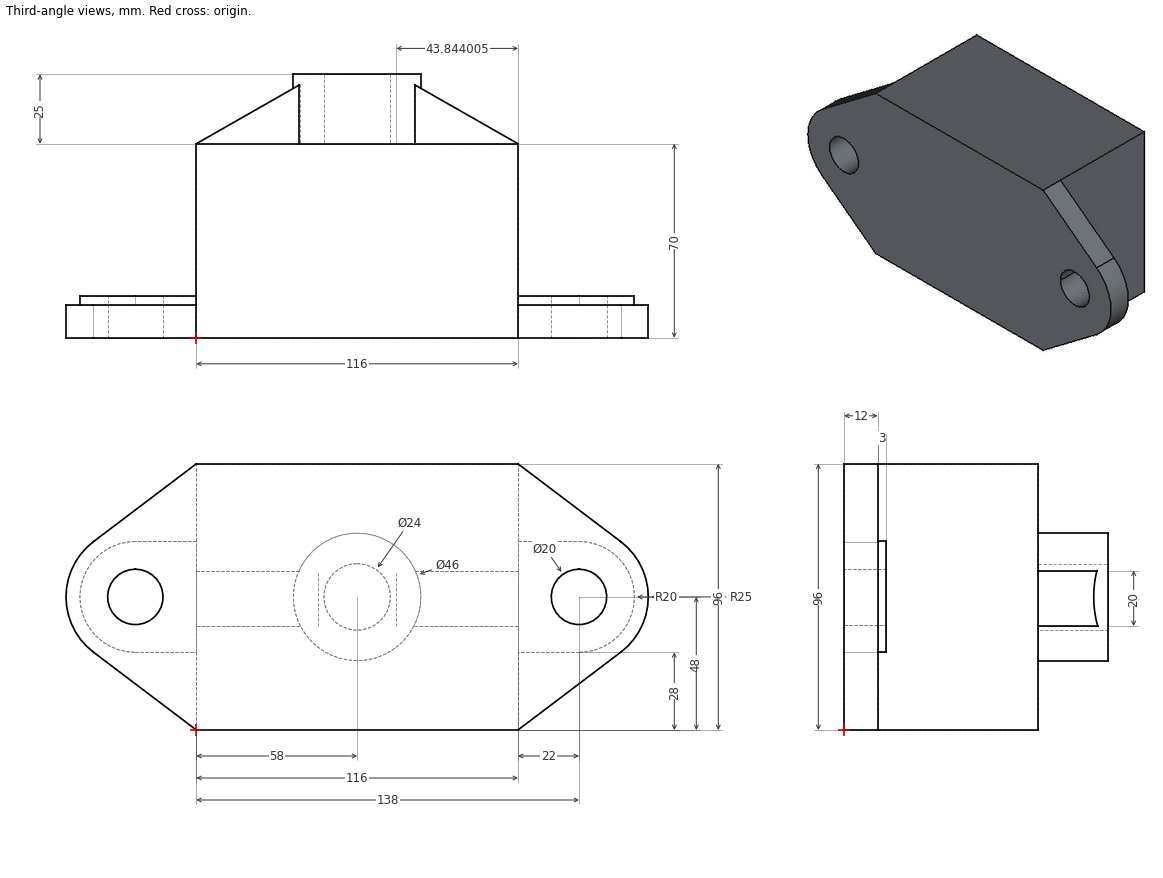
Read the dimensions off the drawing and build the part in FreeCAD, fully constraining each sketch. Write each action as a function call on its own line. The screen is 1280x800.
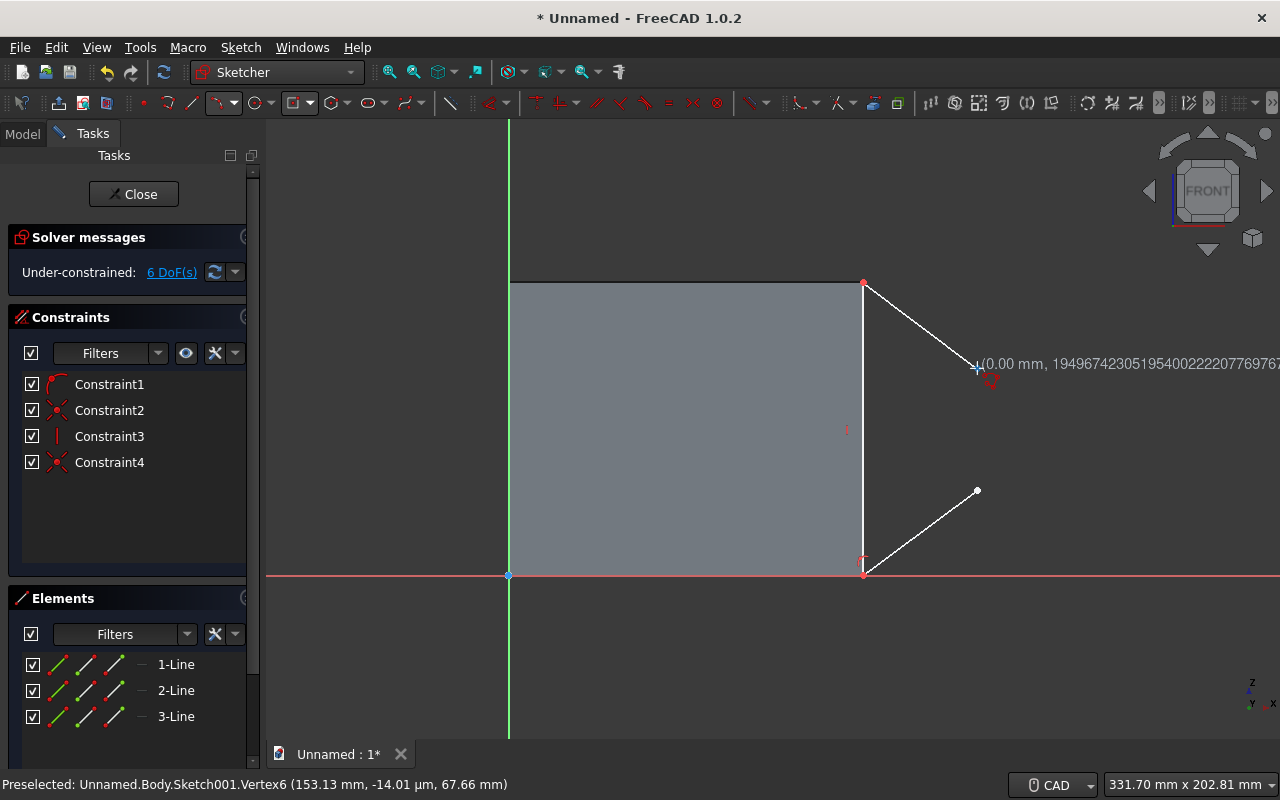
click(218, 104)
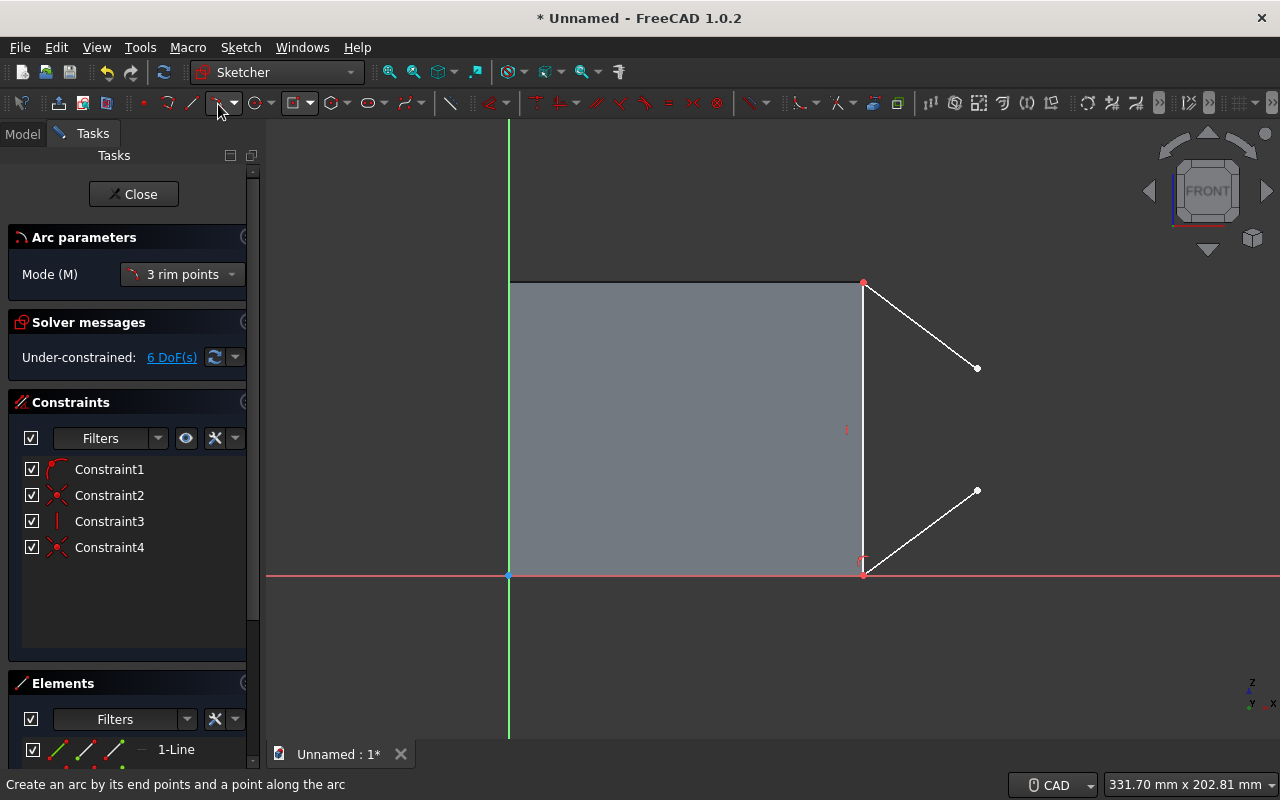
click(977, 369)
click(977, 491)
click(1007, 429)
key(Escape)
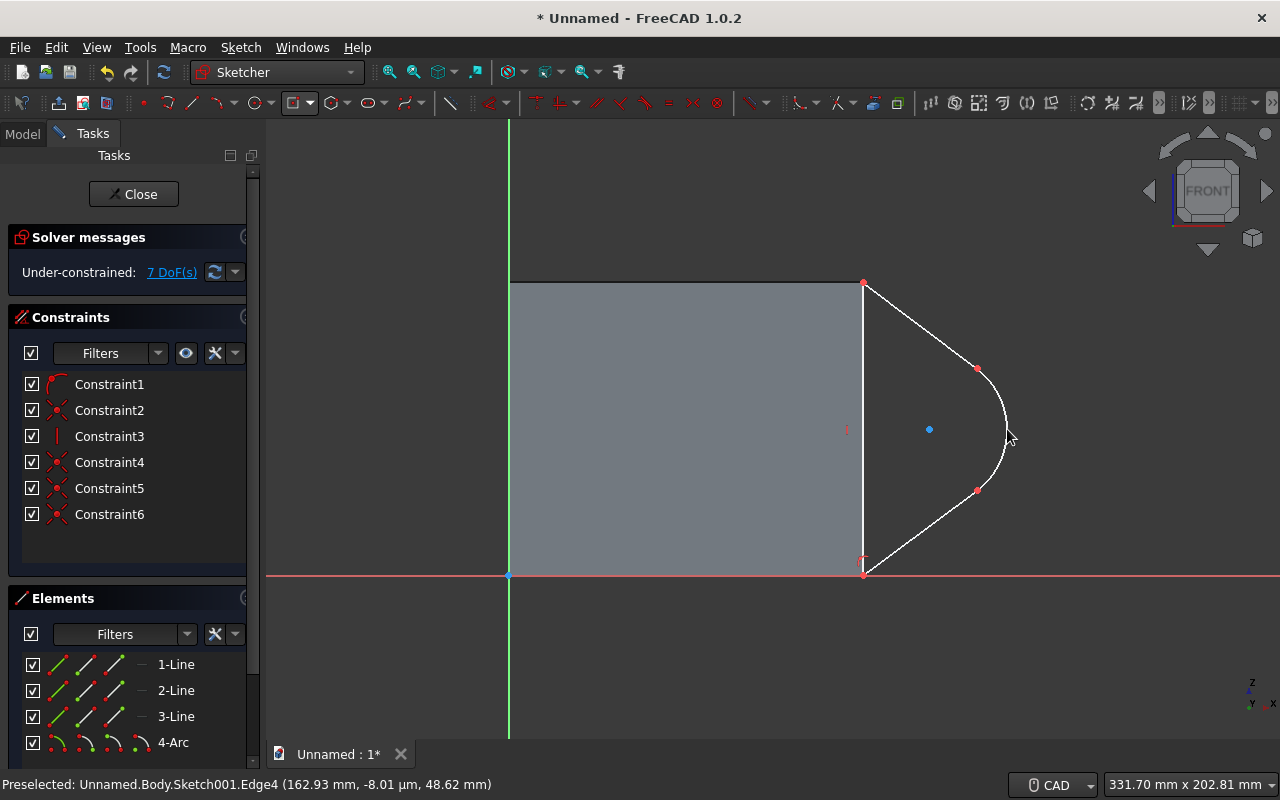
click(943, 516)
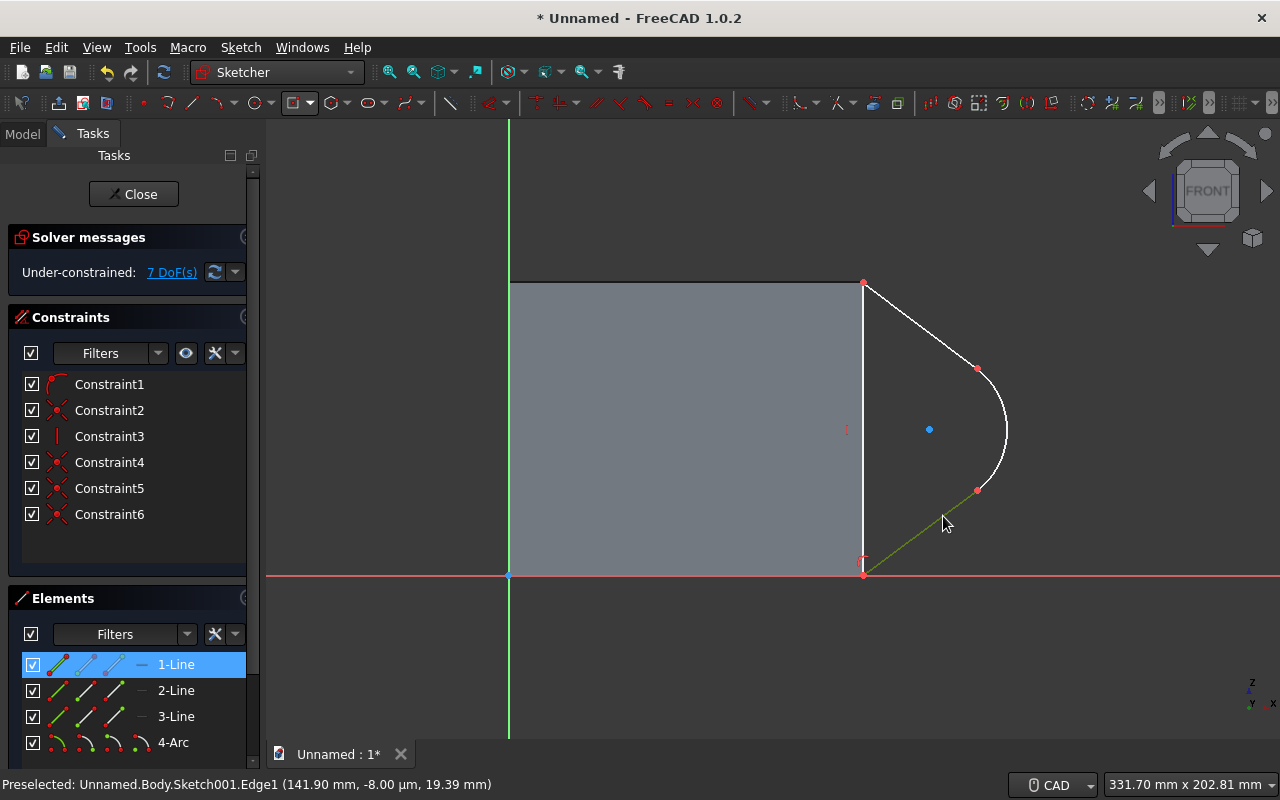
click(1002, 458)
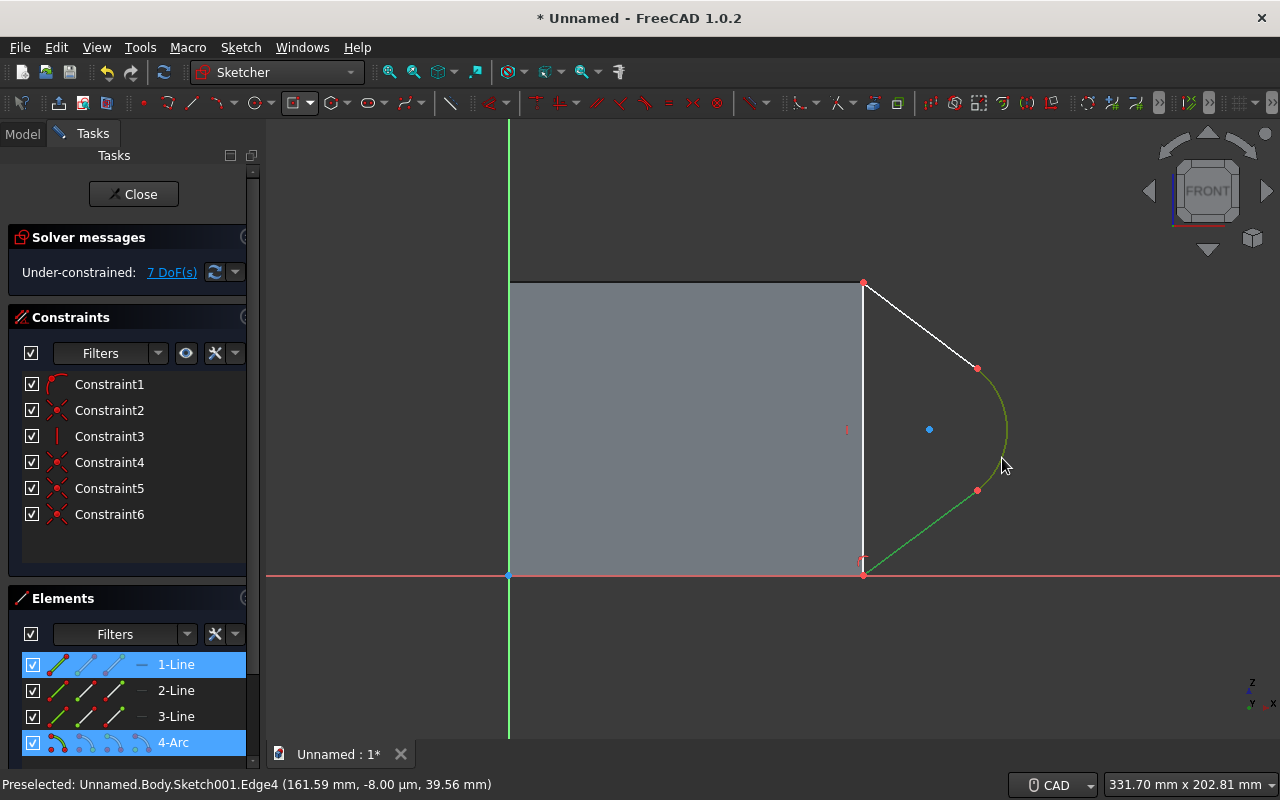
click(646, 104)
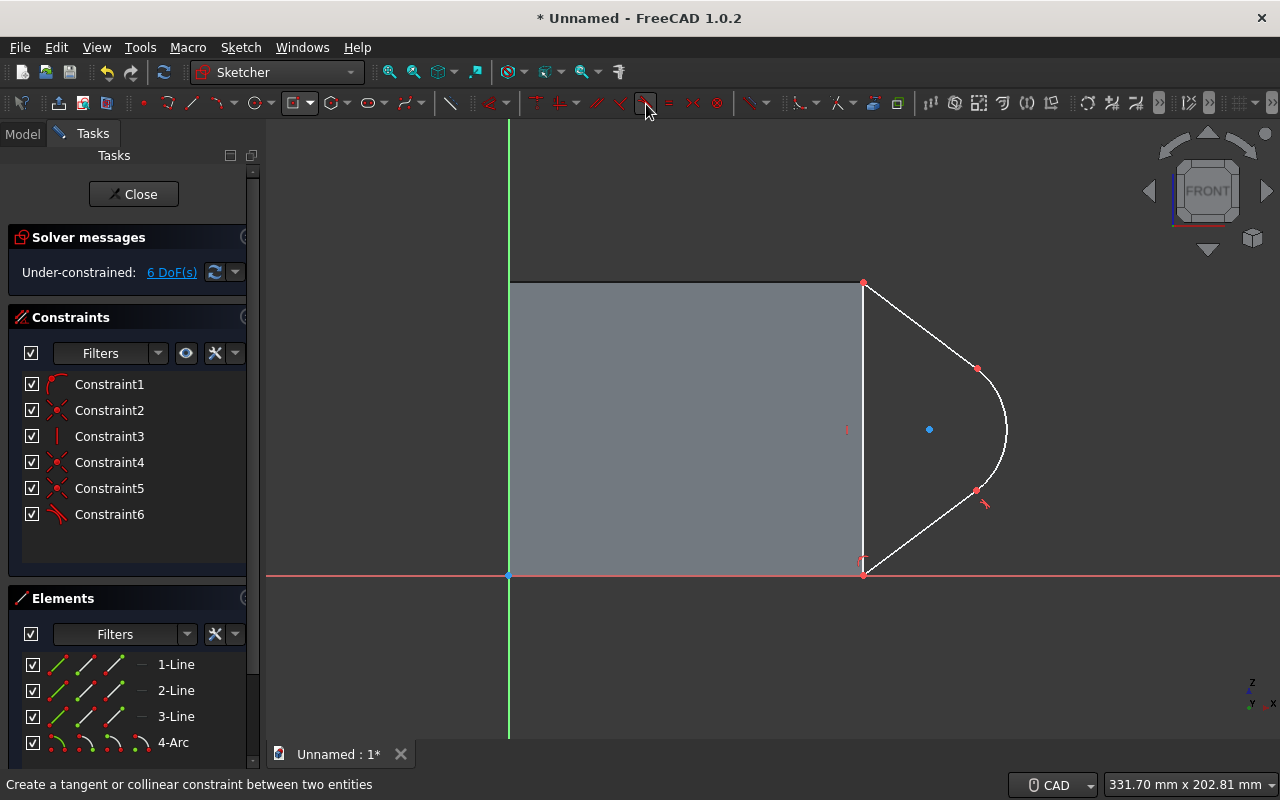
click(897, 309)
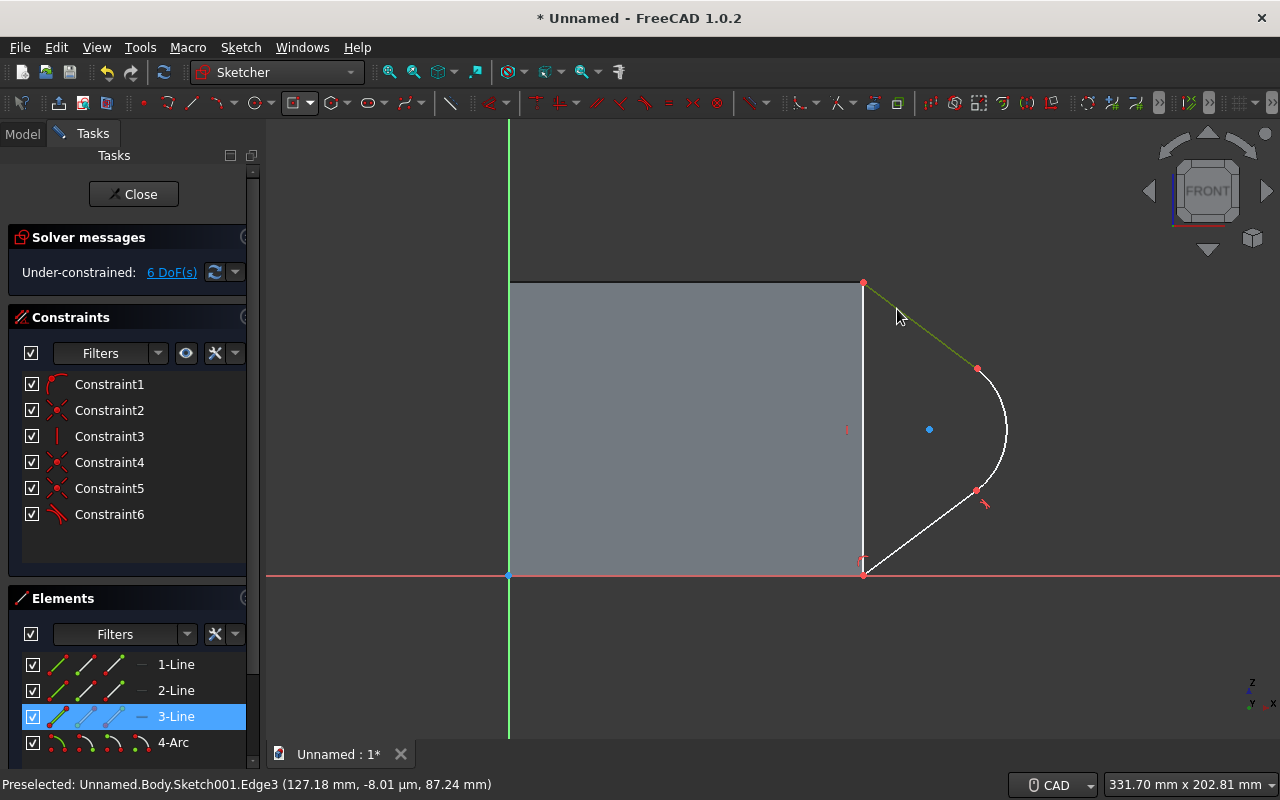
click(1001, 458)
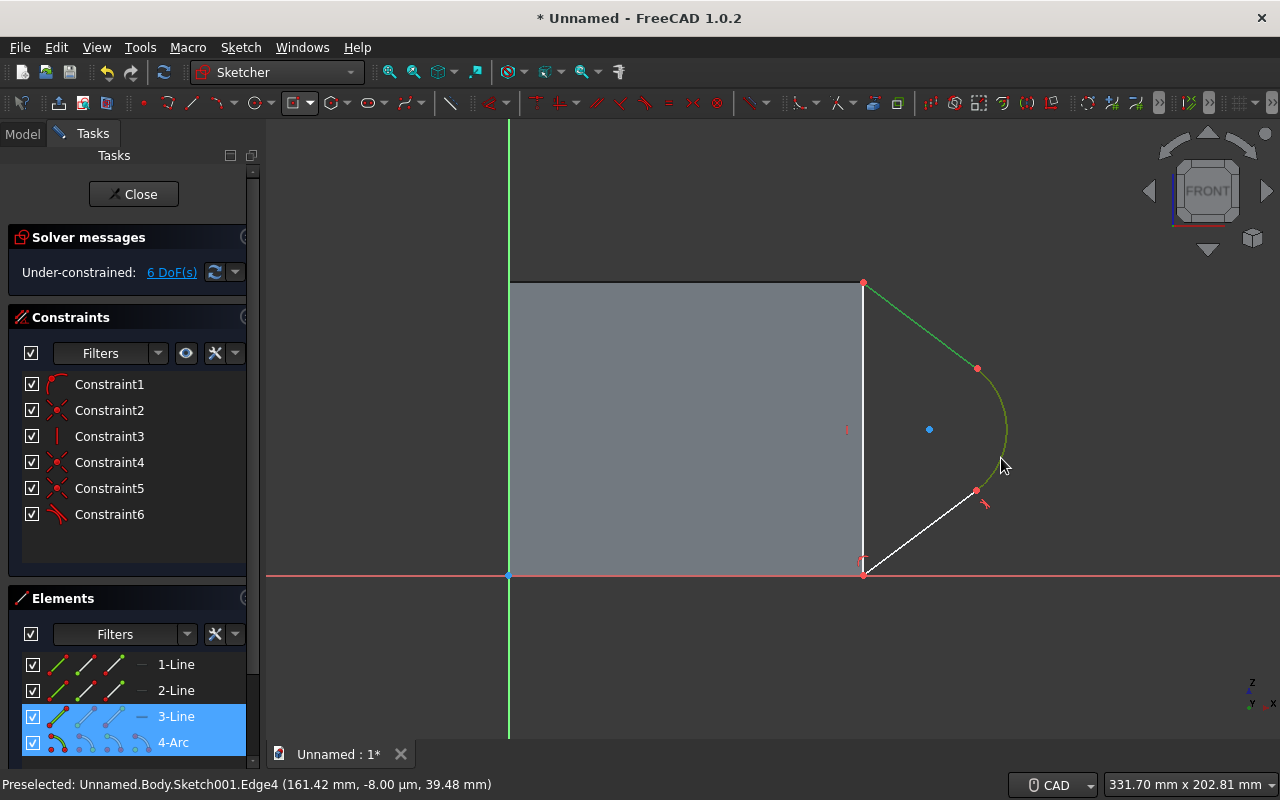
click(646, 104)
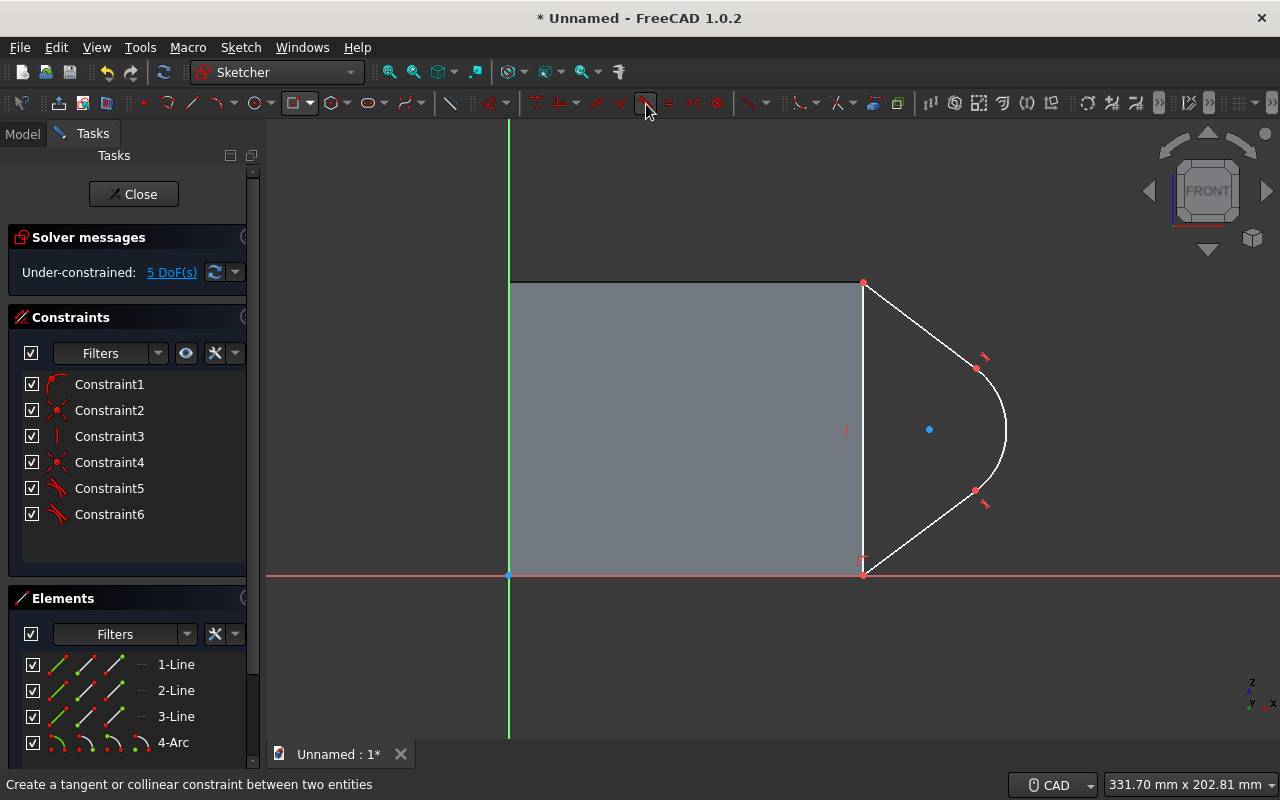
click(490, 104)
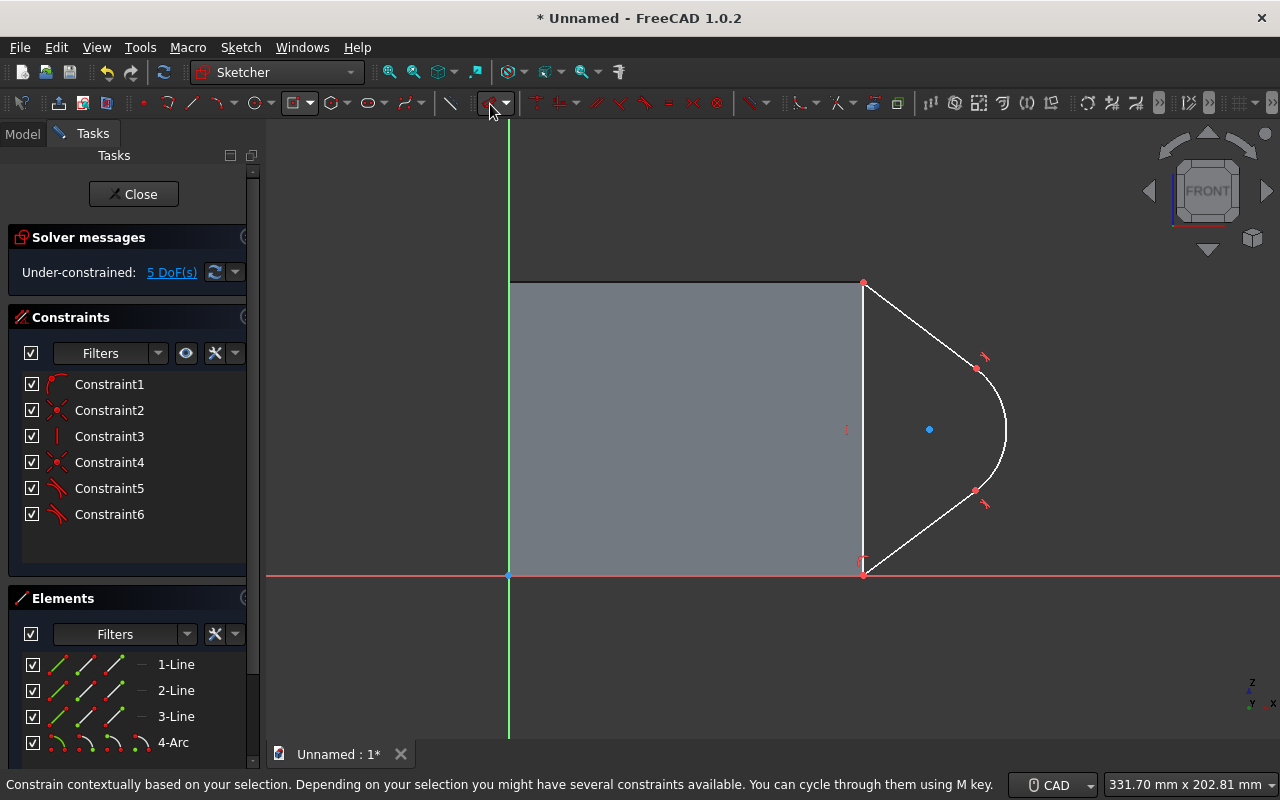
click(1001, 458)
click(1031, 470)